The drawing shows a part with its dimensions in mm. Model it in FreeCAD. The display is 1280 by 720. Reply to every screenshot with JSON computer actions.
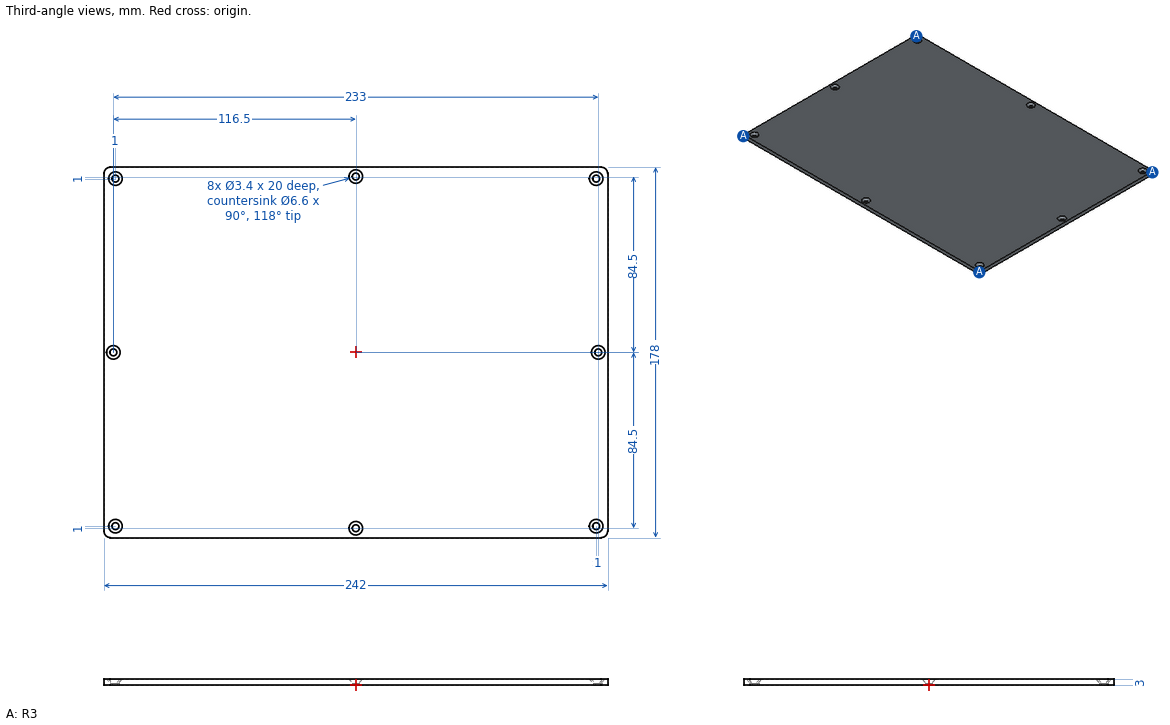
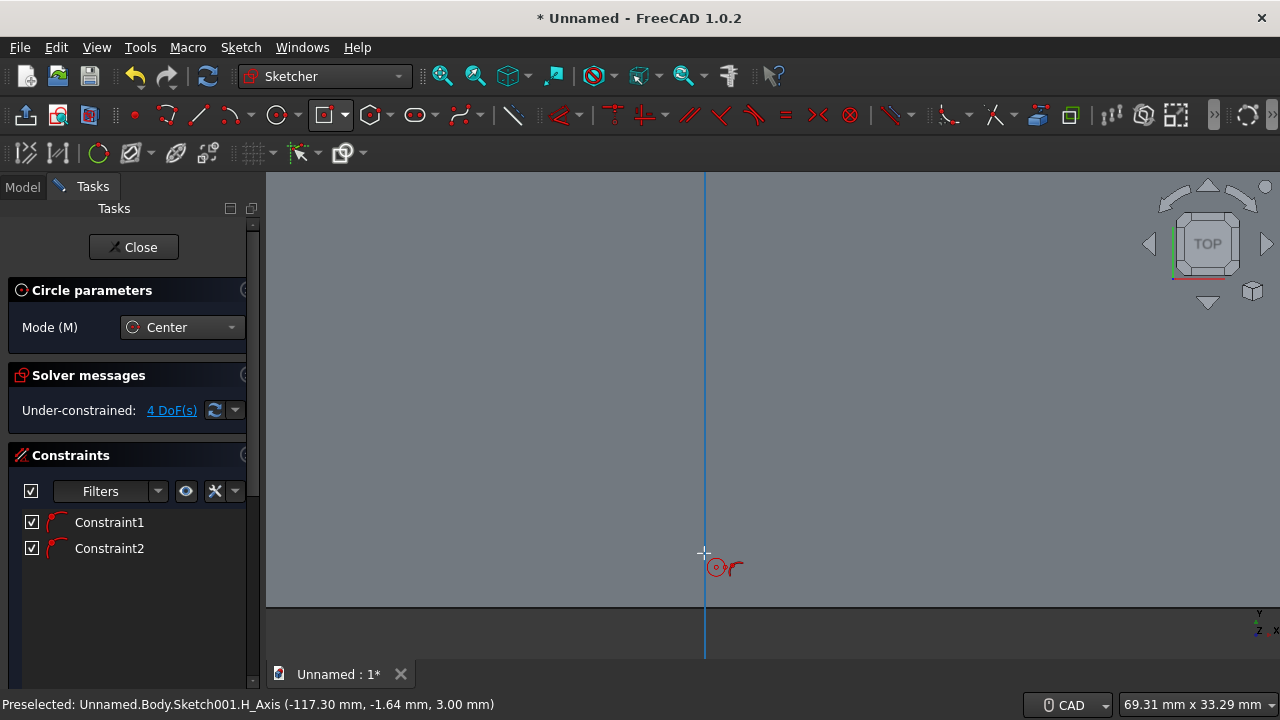
{"action": "scroll", "coordinate": [704, 554], "scroll_direction": "down", "scroll_amount": 11}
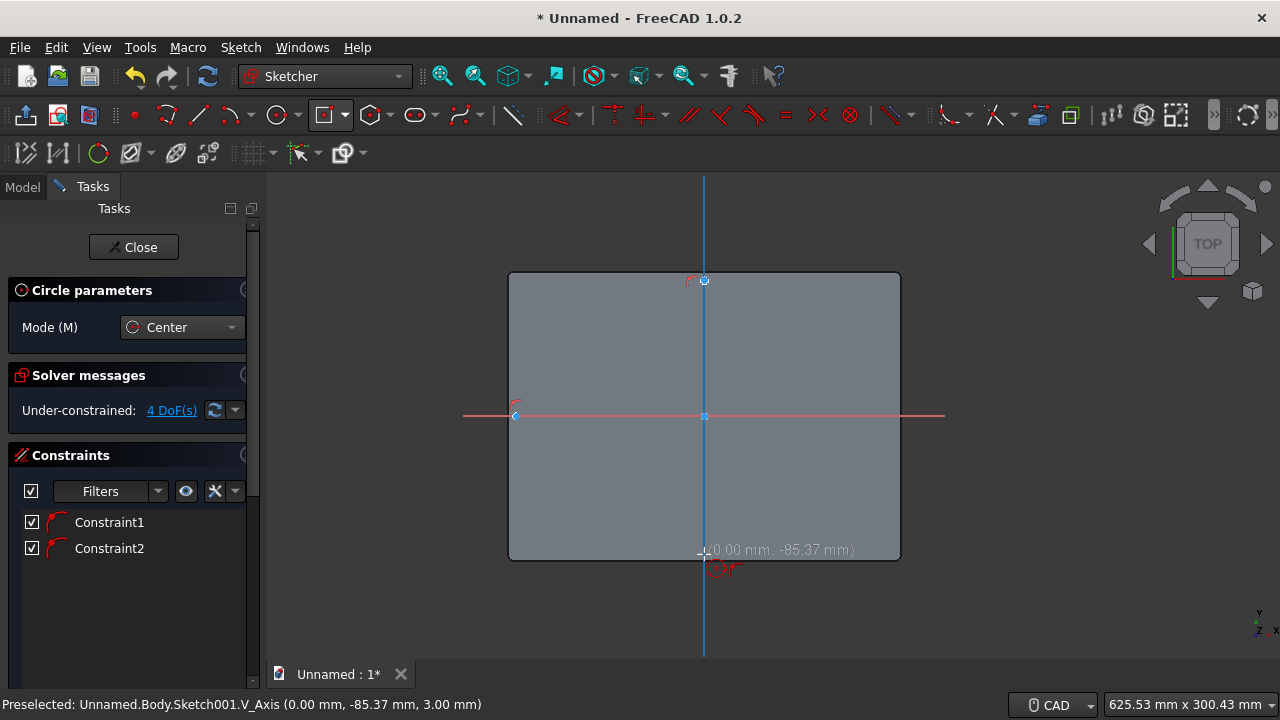
{"action": "left_click", "coordinate": [704, 553]}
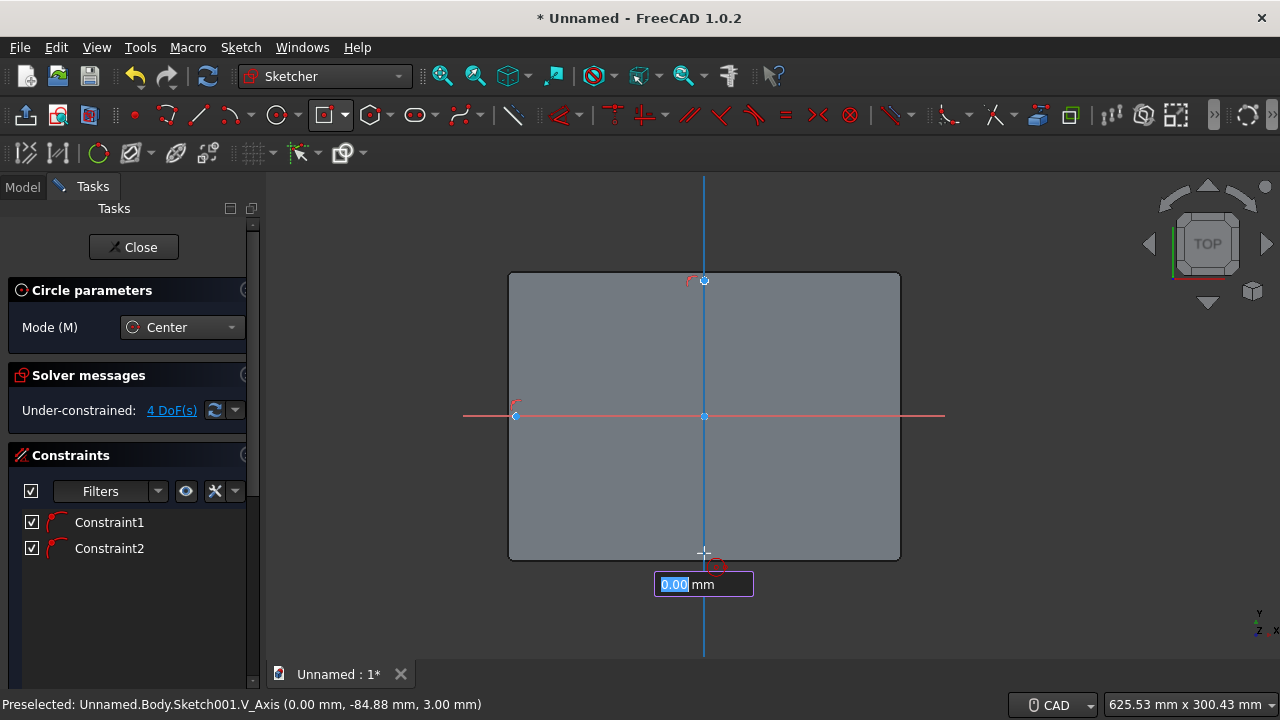
{"action": "scroll", "coordinate": [707, 552], "scroll_direction": "up", "scroll_amount": 10}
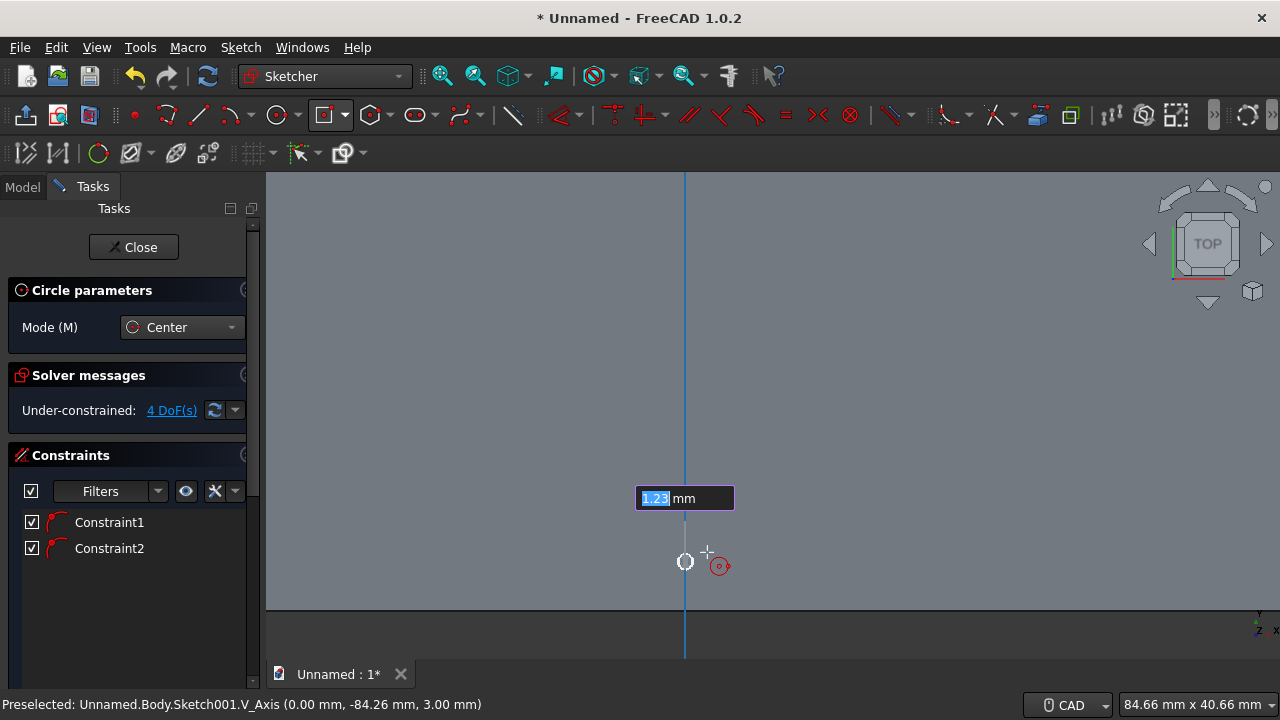
{"action": "left_click", "coordinate": [705, 550]}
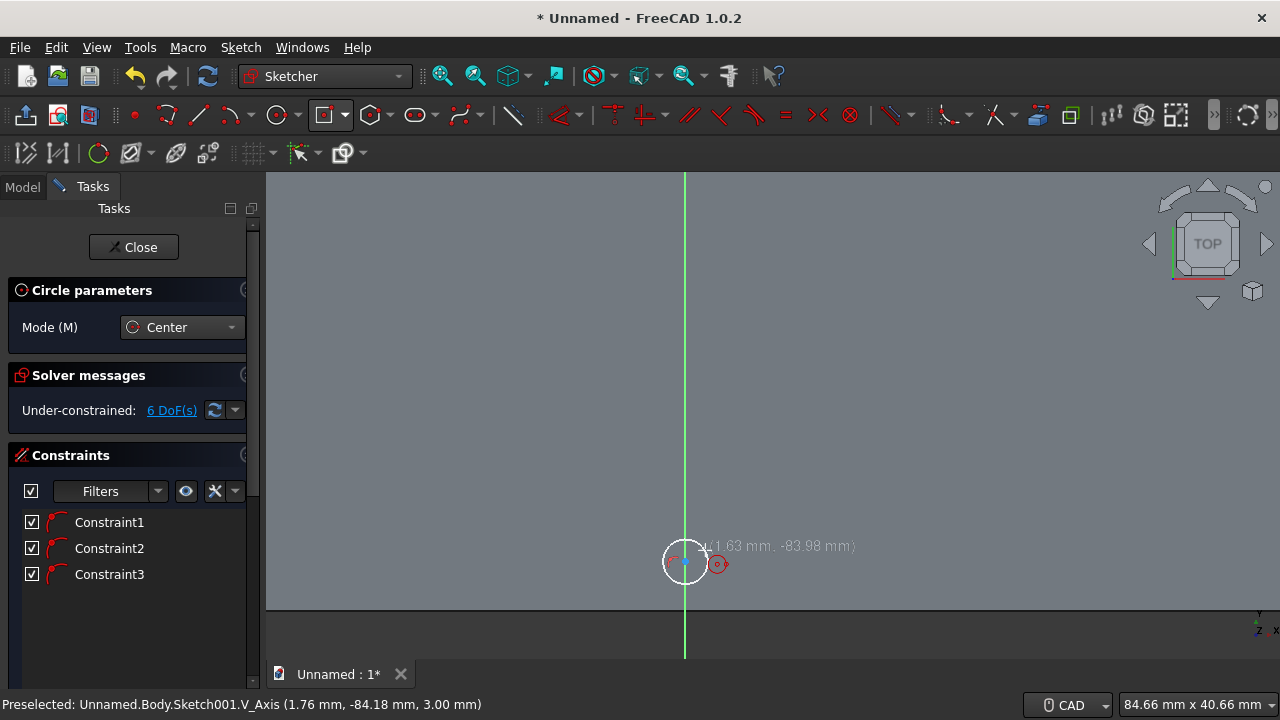
{"action": "scroll", "coordinate": [707, 552], "scroll_direction": "down", "scroll_amount": 10}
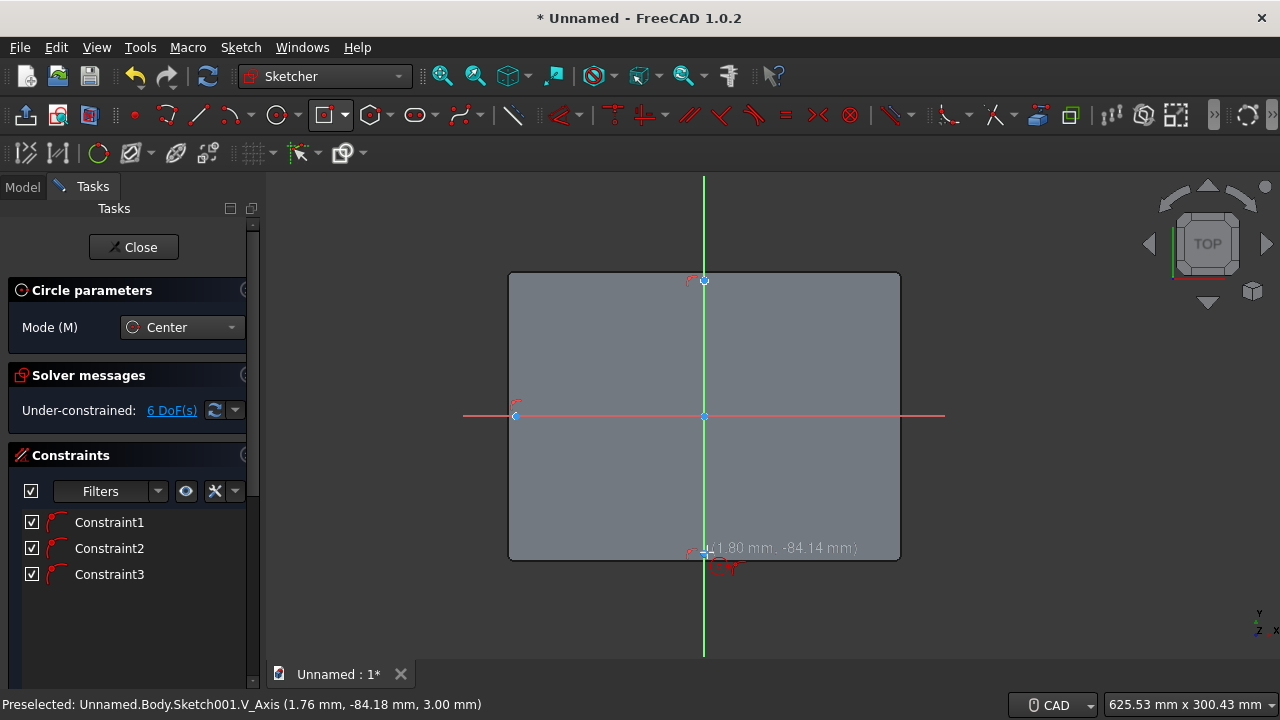
{"action": "scroll", "coordinate": [893, 416], "scroll_direction": "up", "scroll_amount": 11}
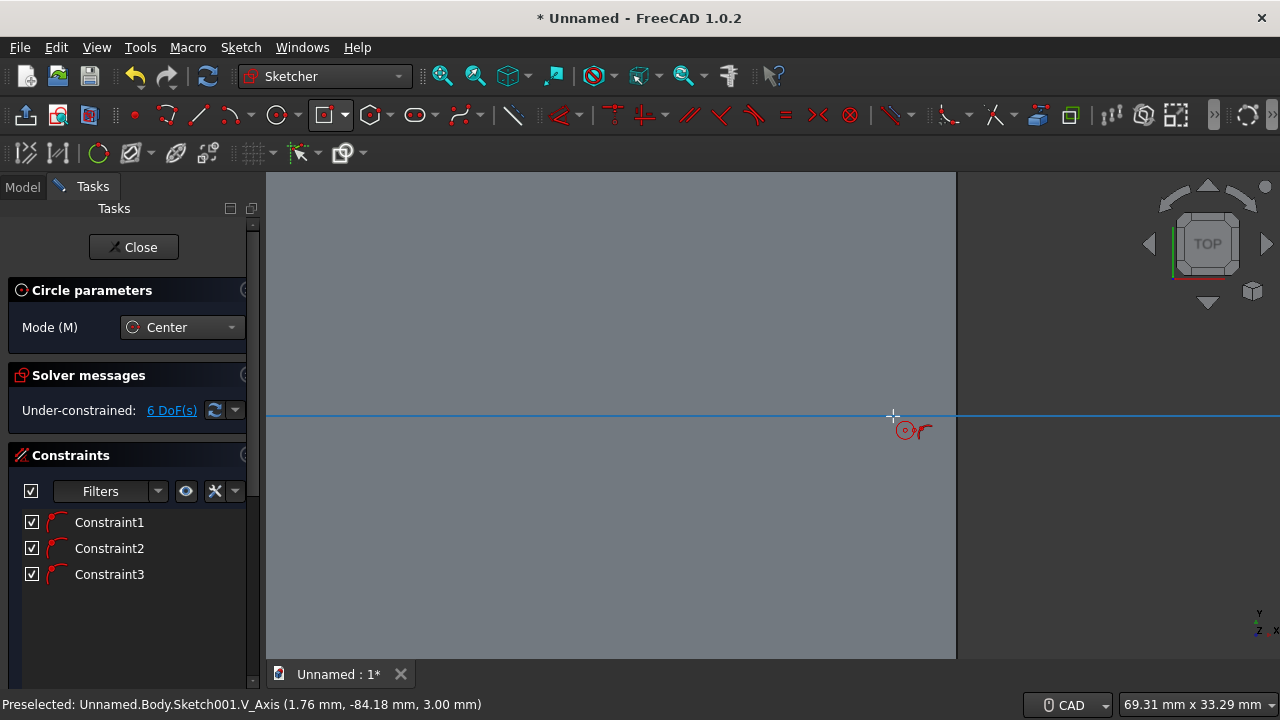
{"action": "scroll", "coordinate": [894, 415], "scroll_direction": "down", "scroll_amount": 11}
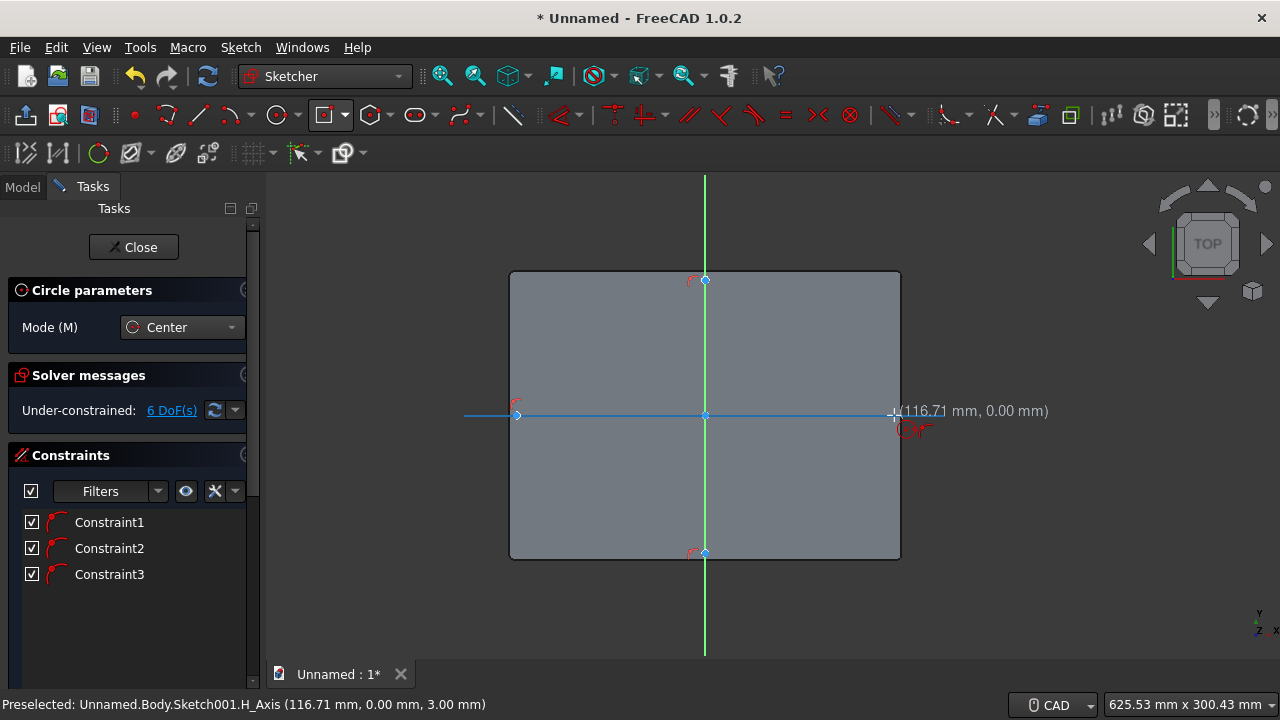
{"action": "left_click", "coordinate": [894, 416]}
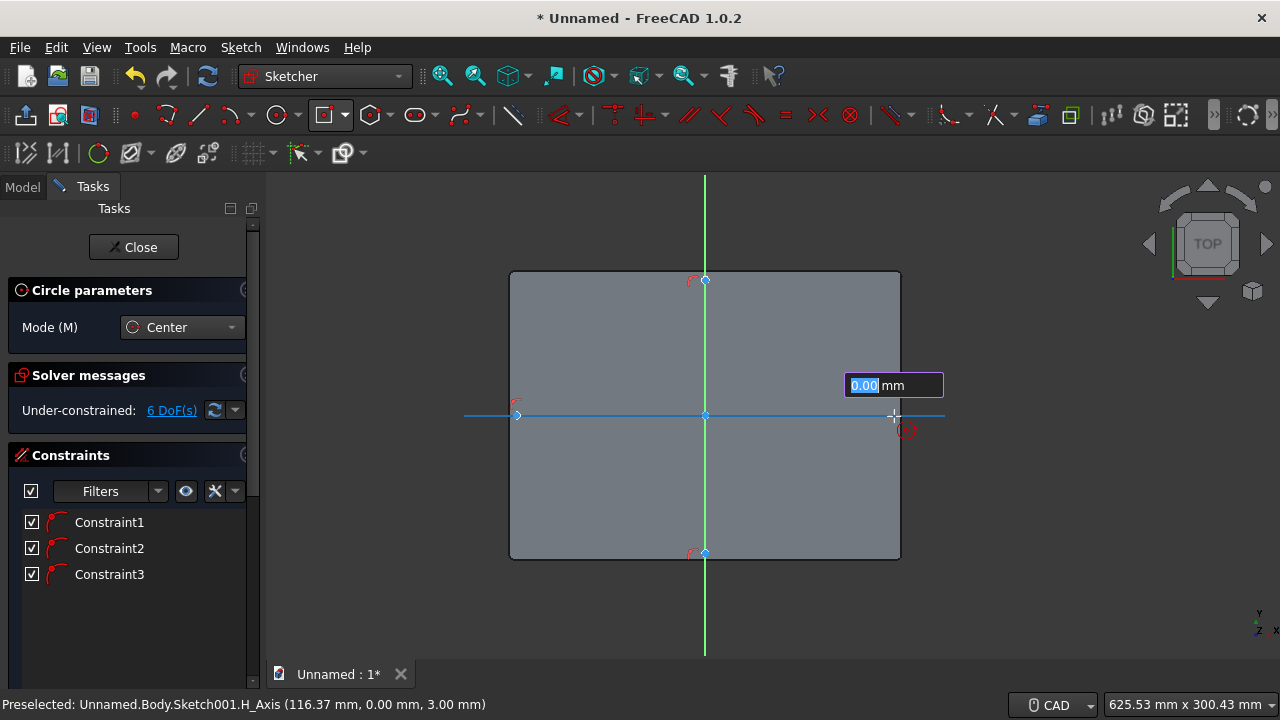
{"action": "scroll", "coordinate": [893, 418], "scroll_direction": "up", "scroll_amount": 10}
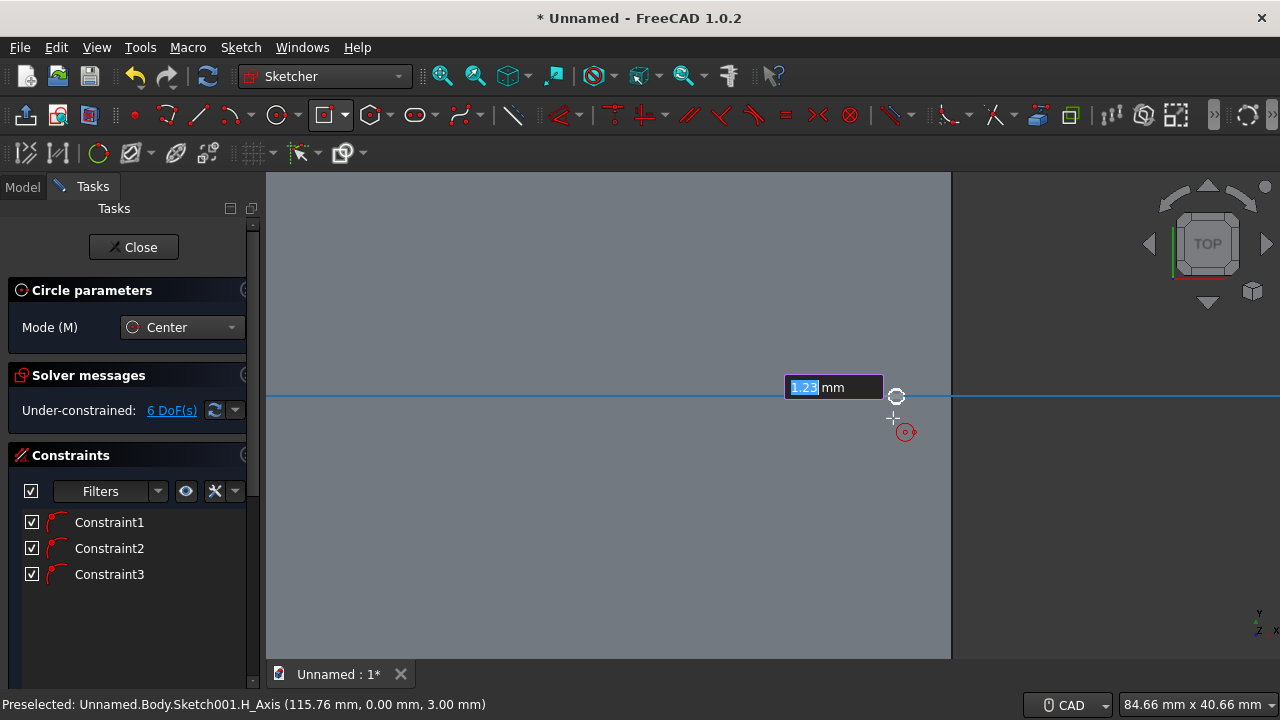
{"action": "left_click", "coordinate": [891, 416]}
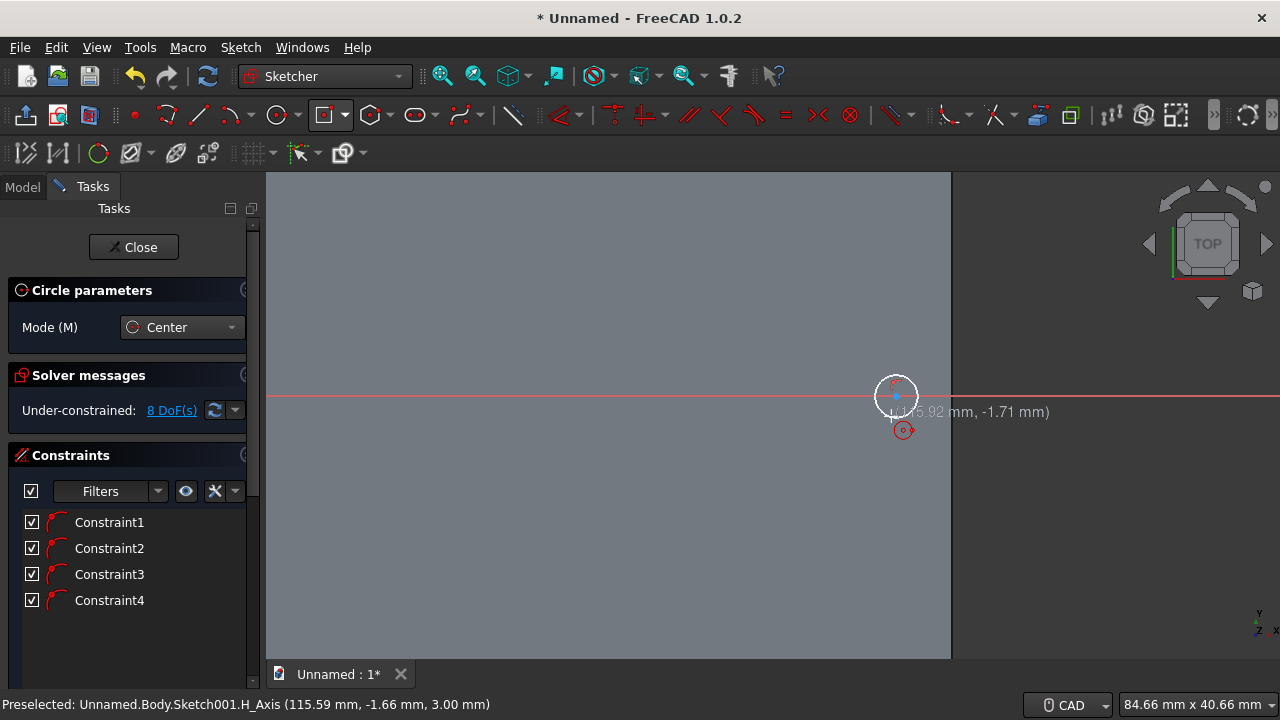
{"action": "scroll", "coordinate": [893, 418], "scroll_direction": "down", "scroll_amount": 10}